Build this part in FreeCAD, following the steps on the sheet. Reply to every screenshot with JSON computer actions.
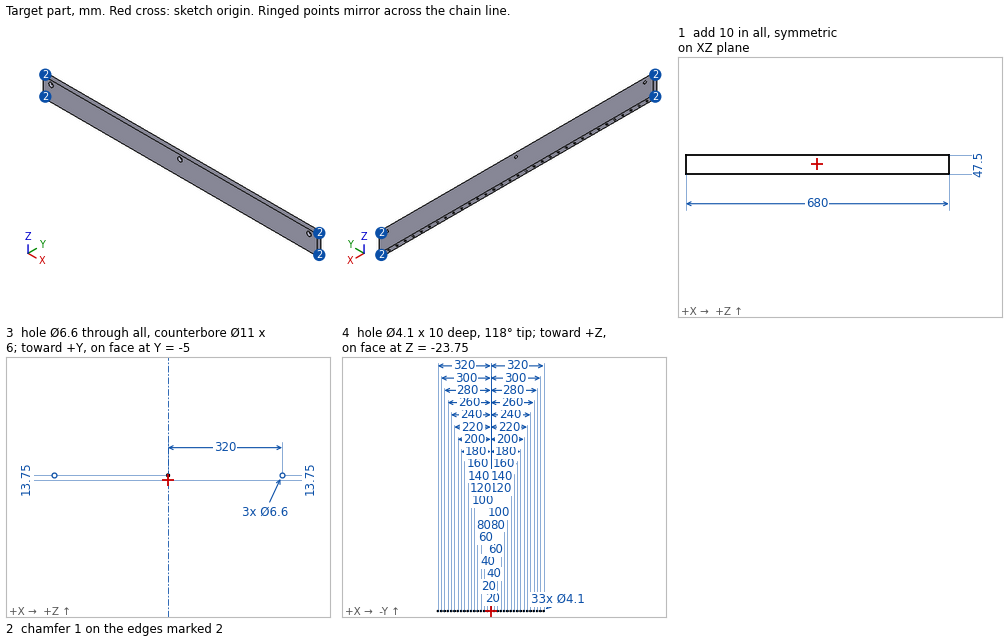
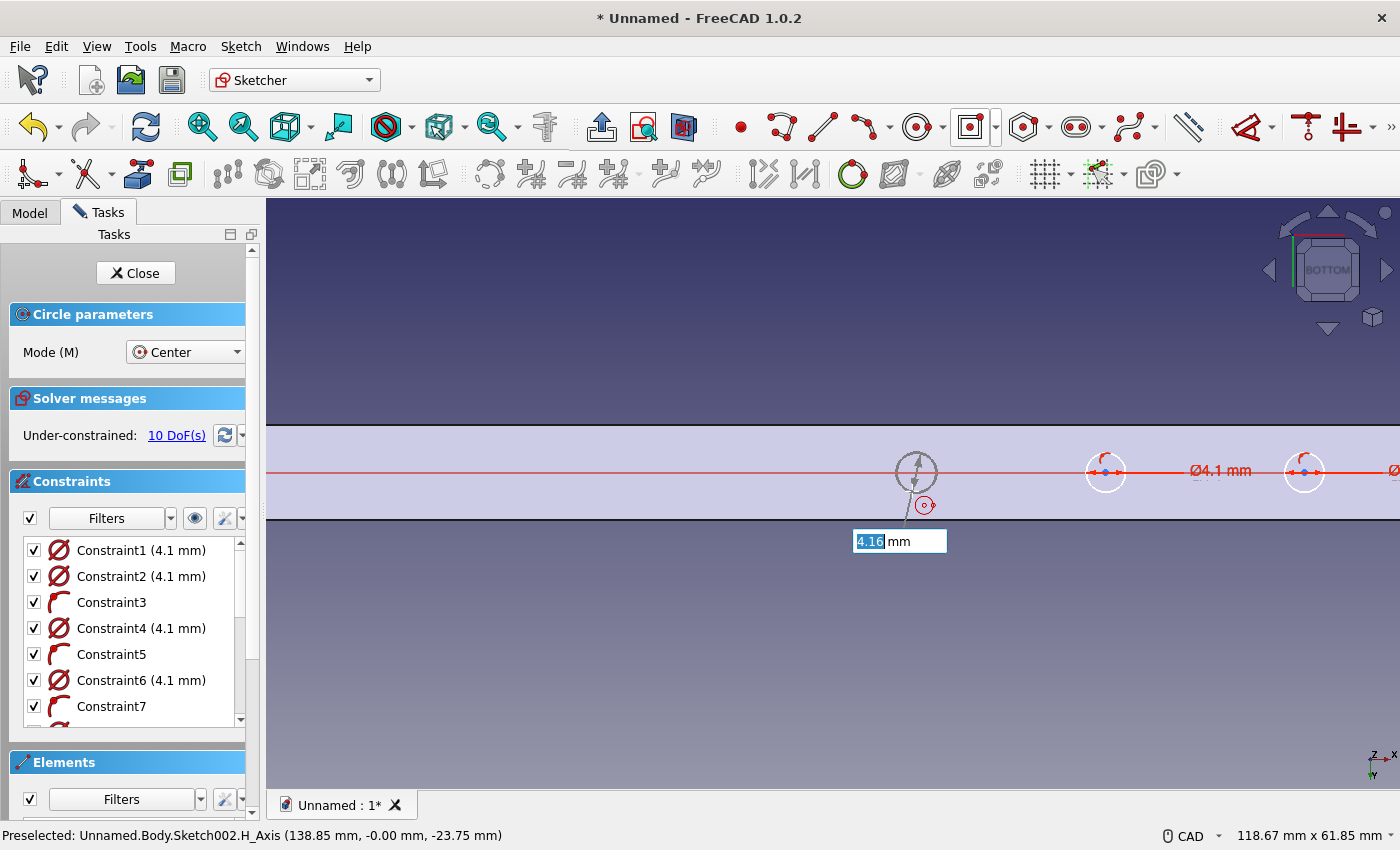
{"action": "type", "text": "4.1"}
{"action": "key", "text": "Return"}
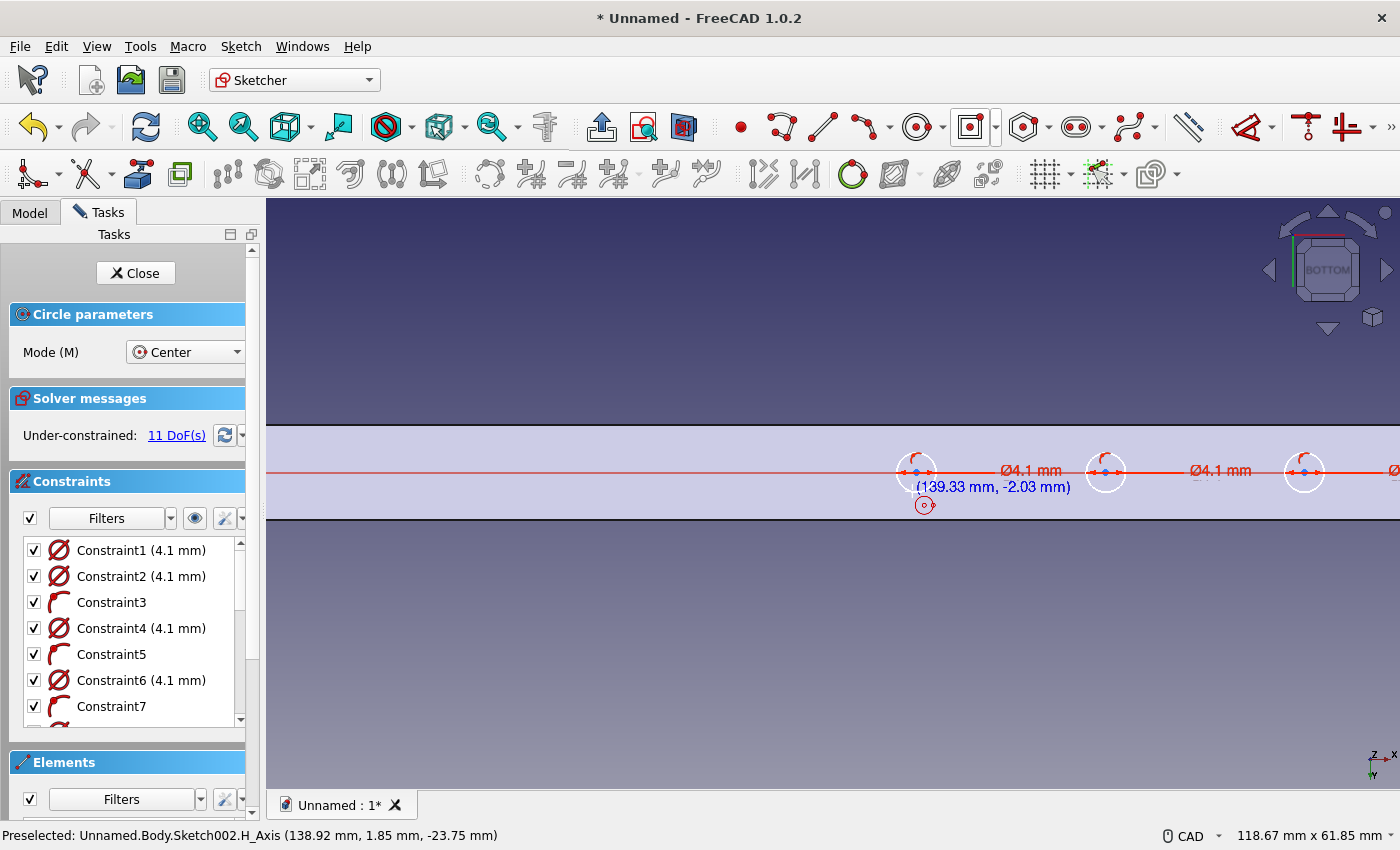
{"action": "scroll", "coordinate": [912, 496], "scroll_direction": "down", "scroll_amount": 11}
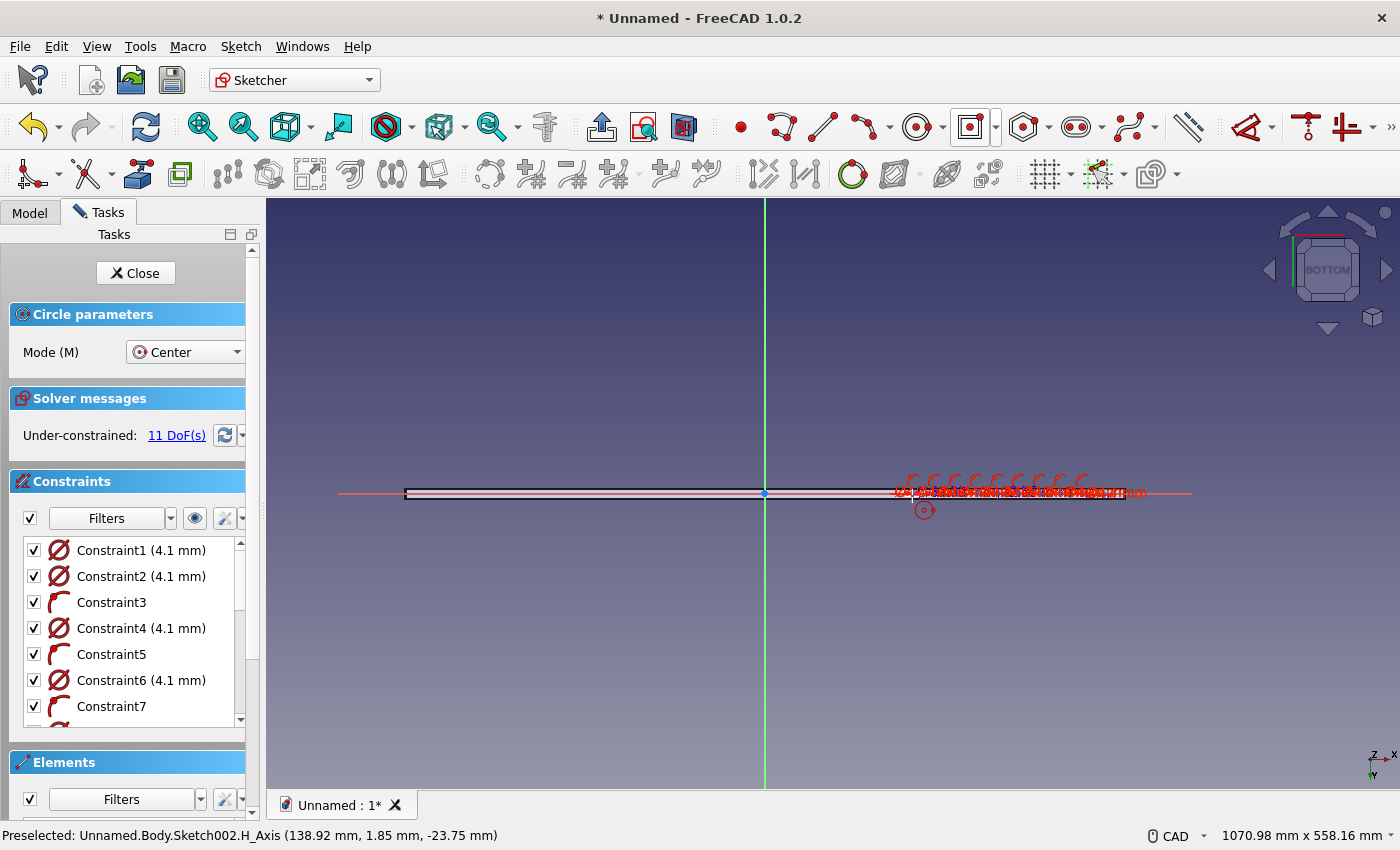
{"action": "left_click", "coordinate": [892, 494]}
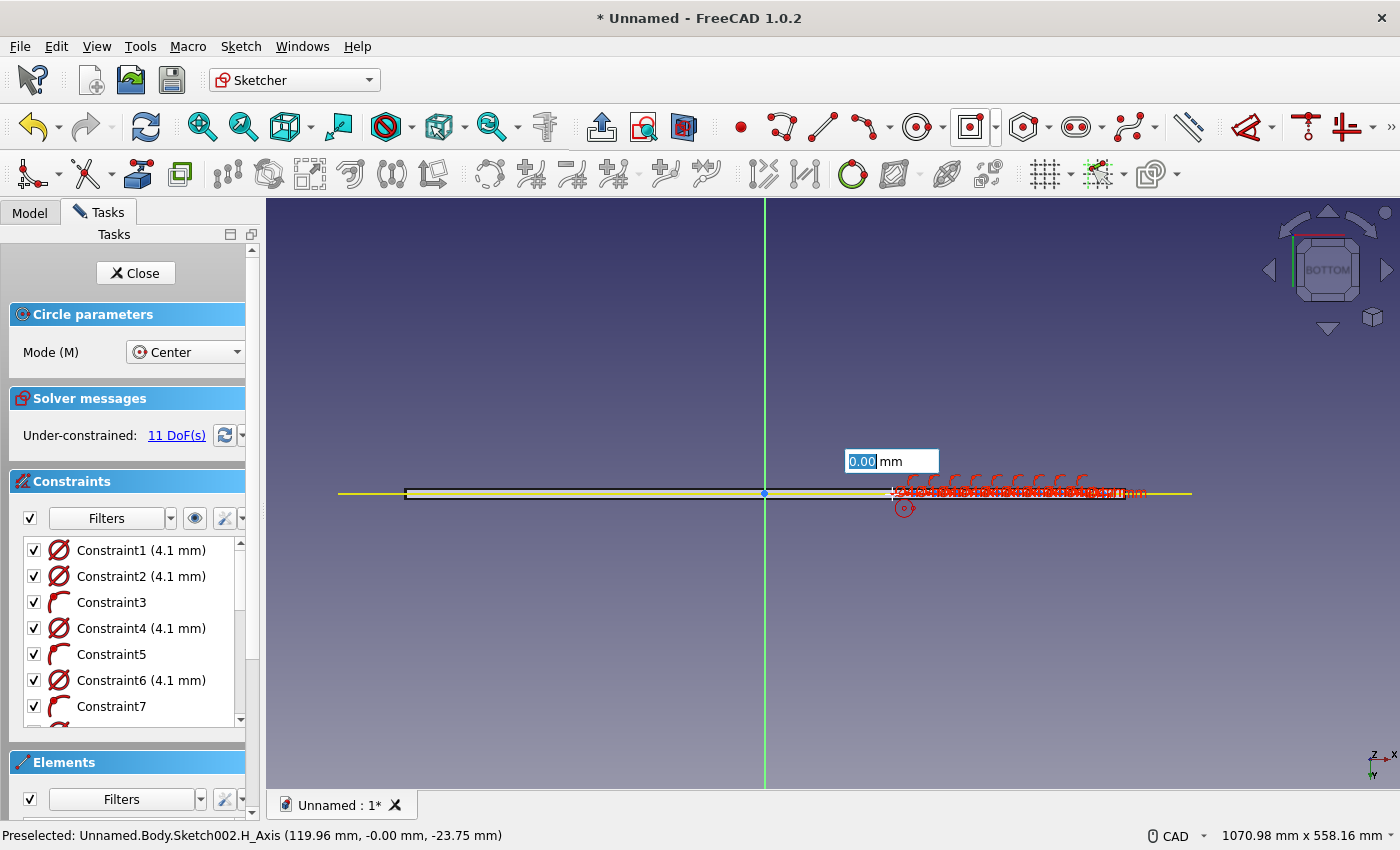
{"action": "scroll", "coordinate": [891, 496], "scroll_direction": "up", "scroll_amount": 11}
{"action": "mouse_move", "coordinate": [889, 491]}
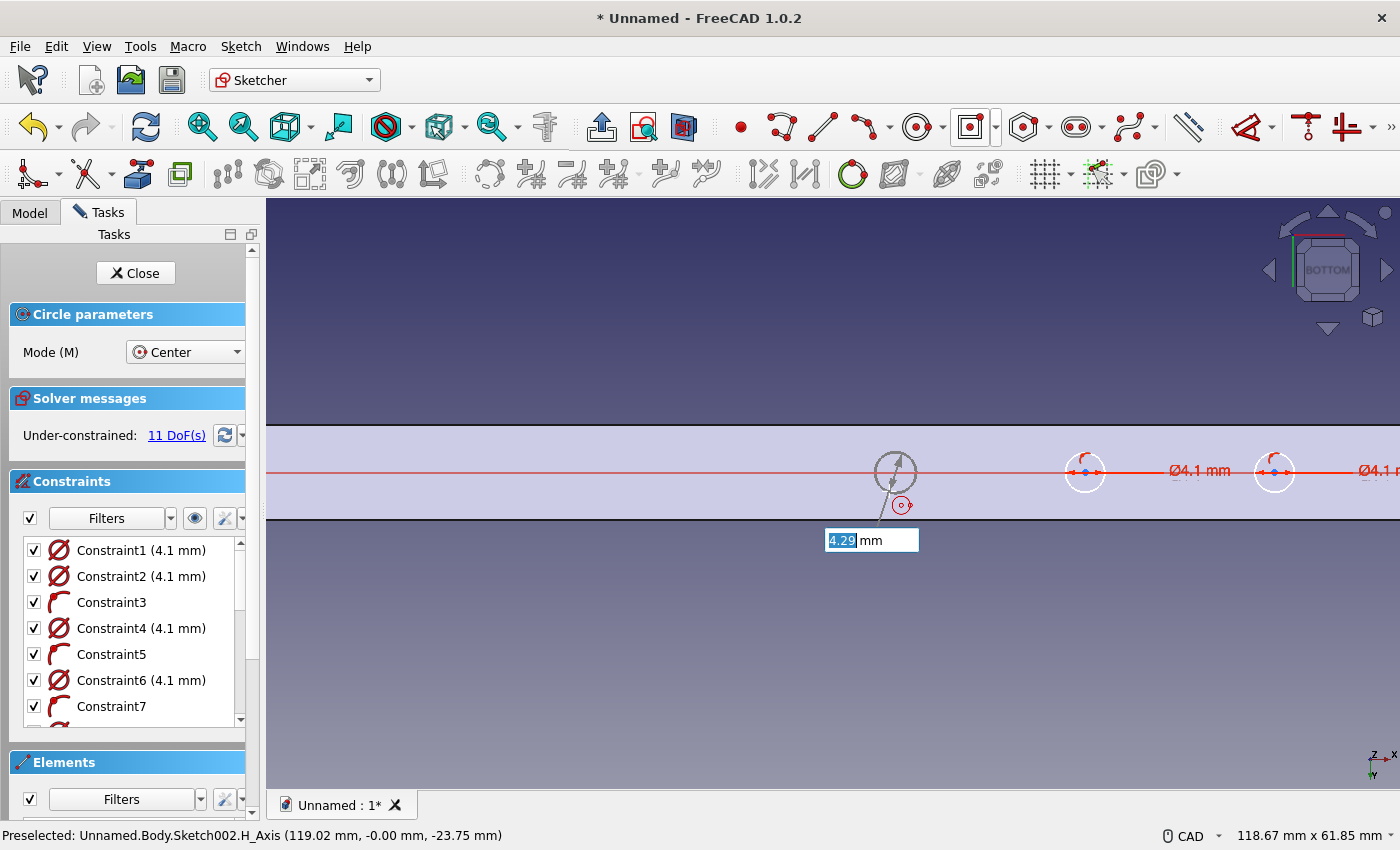
{"action": "type", "text": "4.1"}
{"action": "key", "text": "Return"}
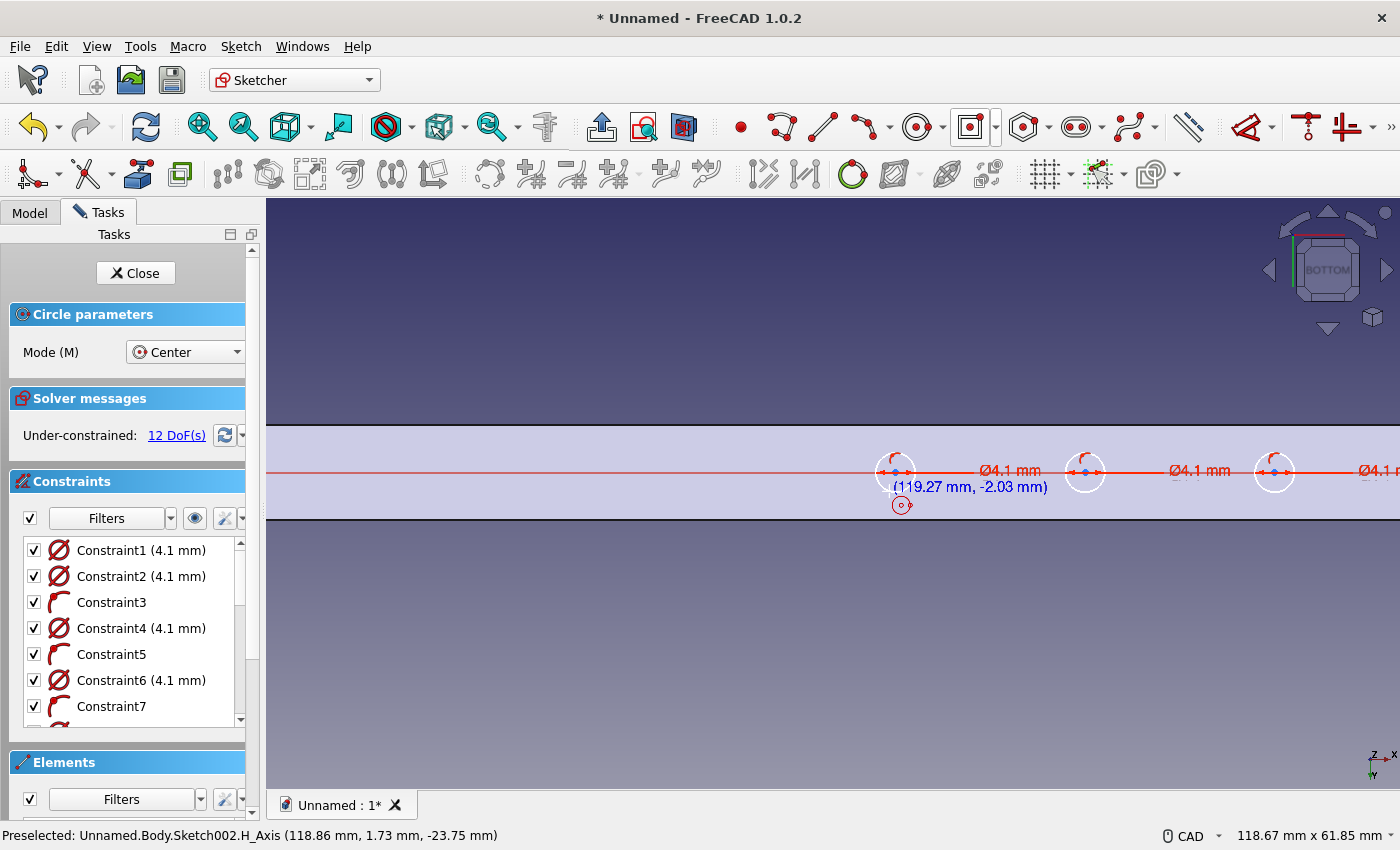
{"action": "scroll", "coordinate": [891, 496], "scroll_direction": "down", "scroll_amount": 11}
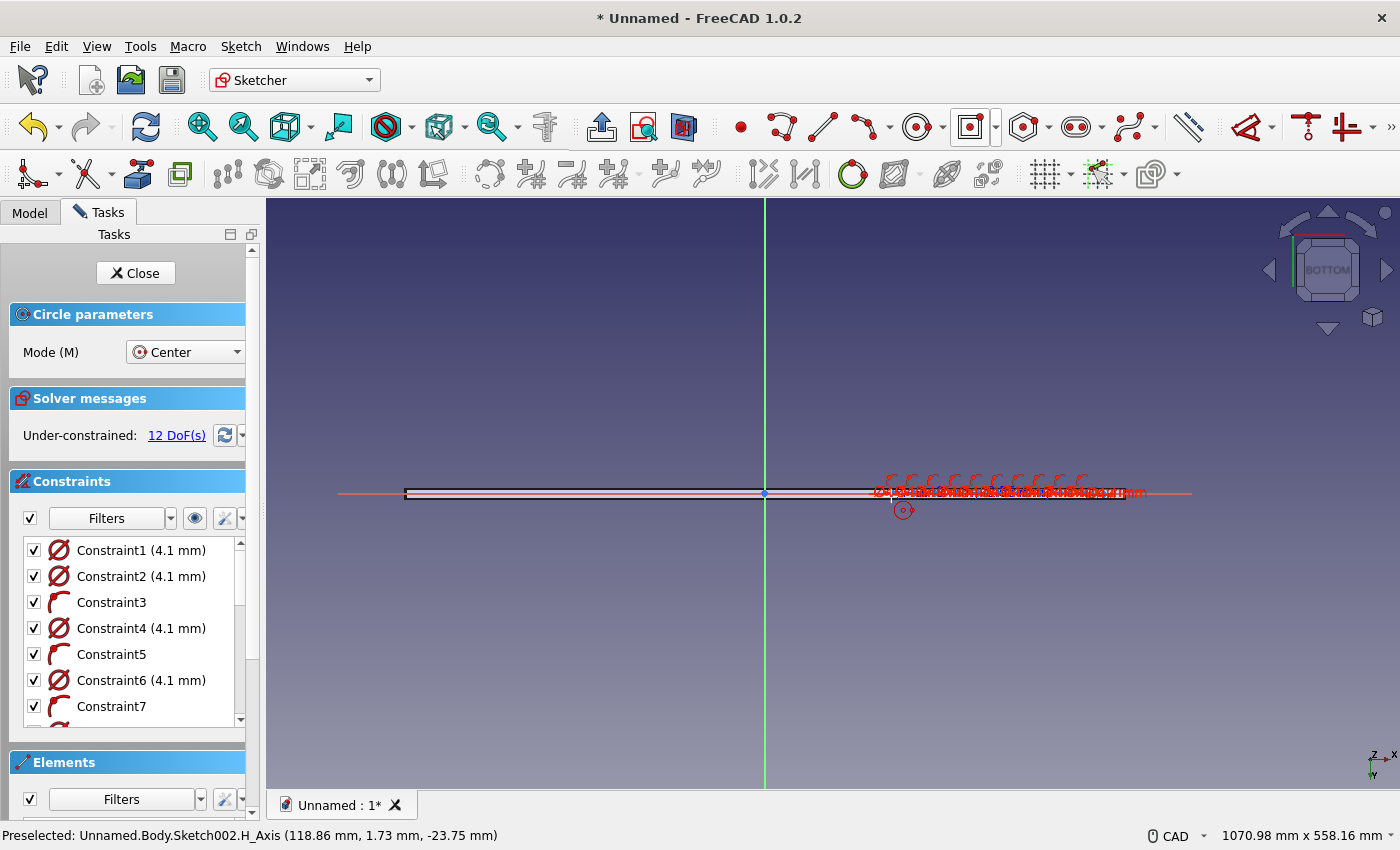
{"action": "left_click", "coordinate": [871, 494]}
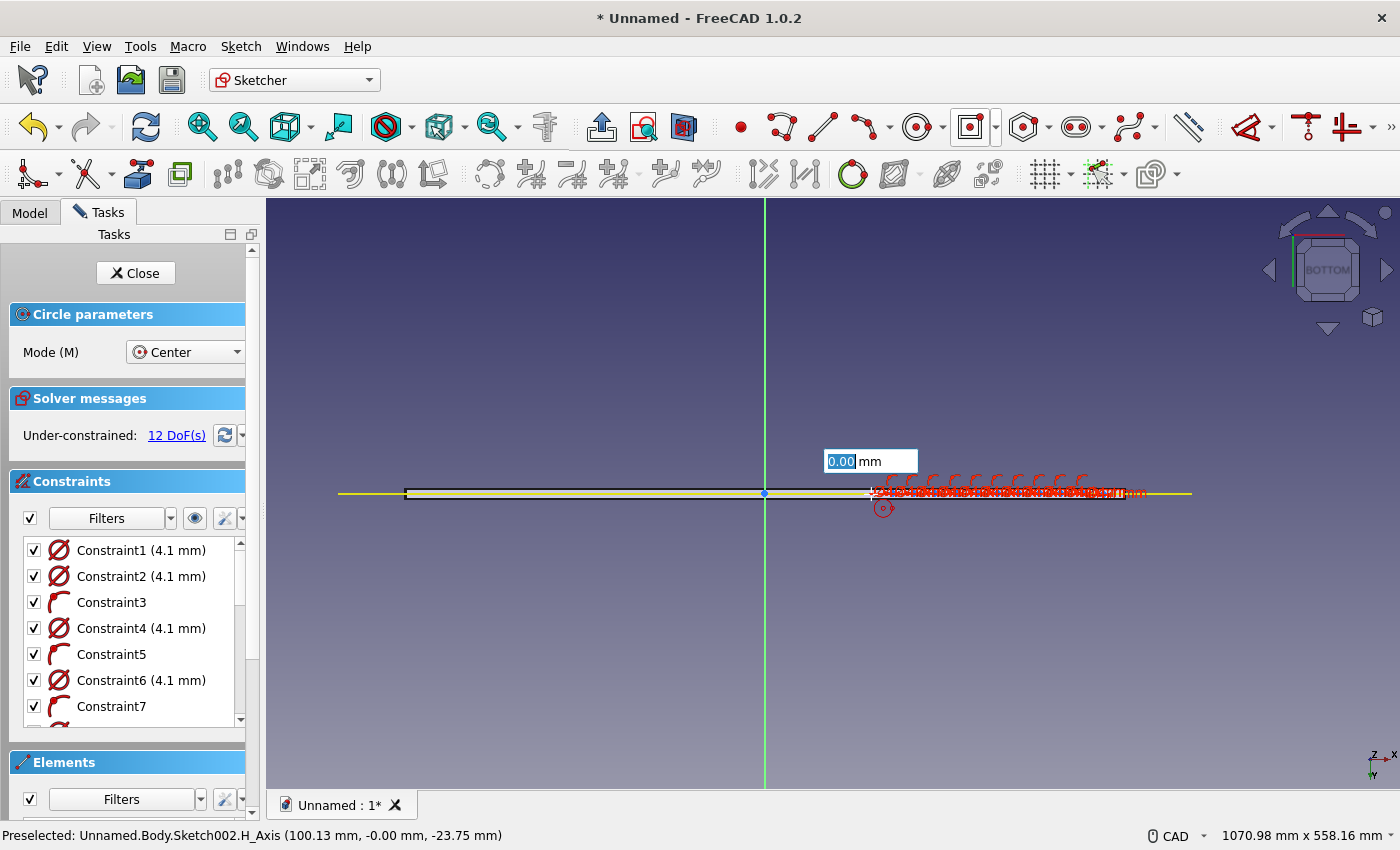
{"action": "scroll", "coordinate": [872, 492], "scroll_direction": "up", "scroll_amount": 11}
{"action": "mouse_move", "coordinate": [864, 486]}